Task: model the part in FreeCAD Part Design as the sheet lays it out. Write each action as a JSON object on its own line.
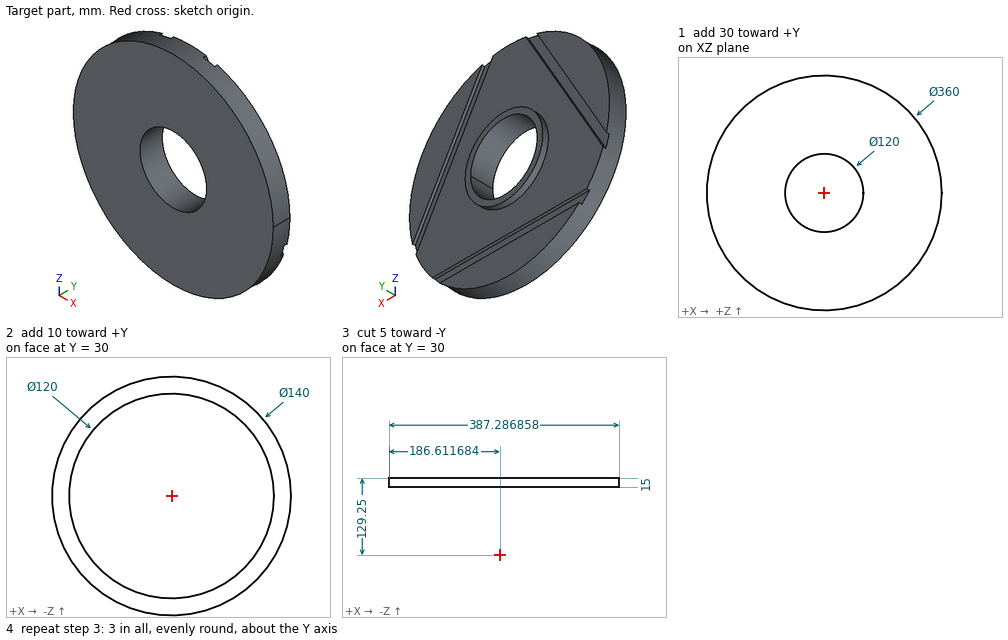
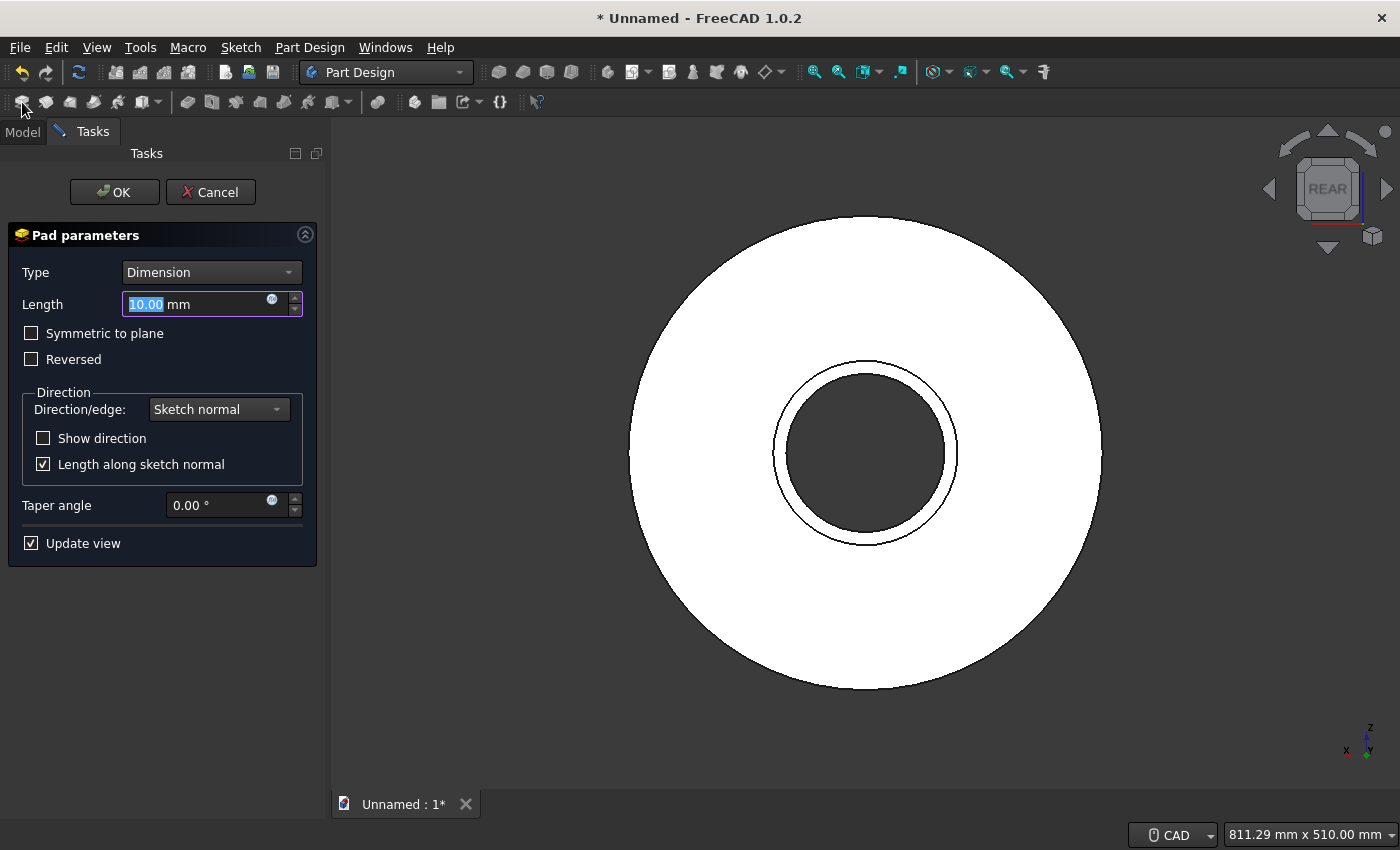
{"action": "type", "text": "10"}
{"action": "key", "text": "Tab"}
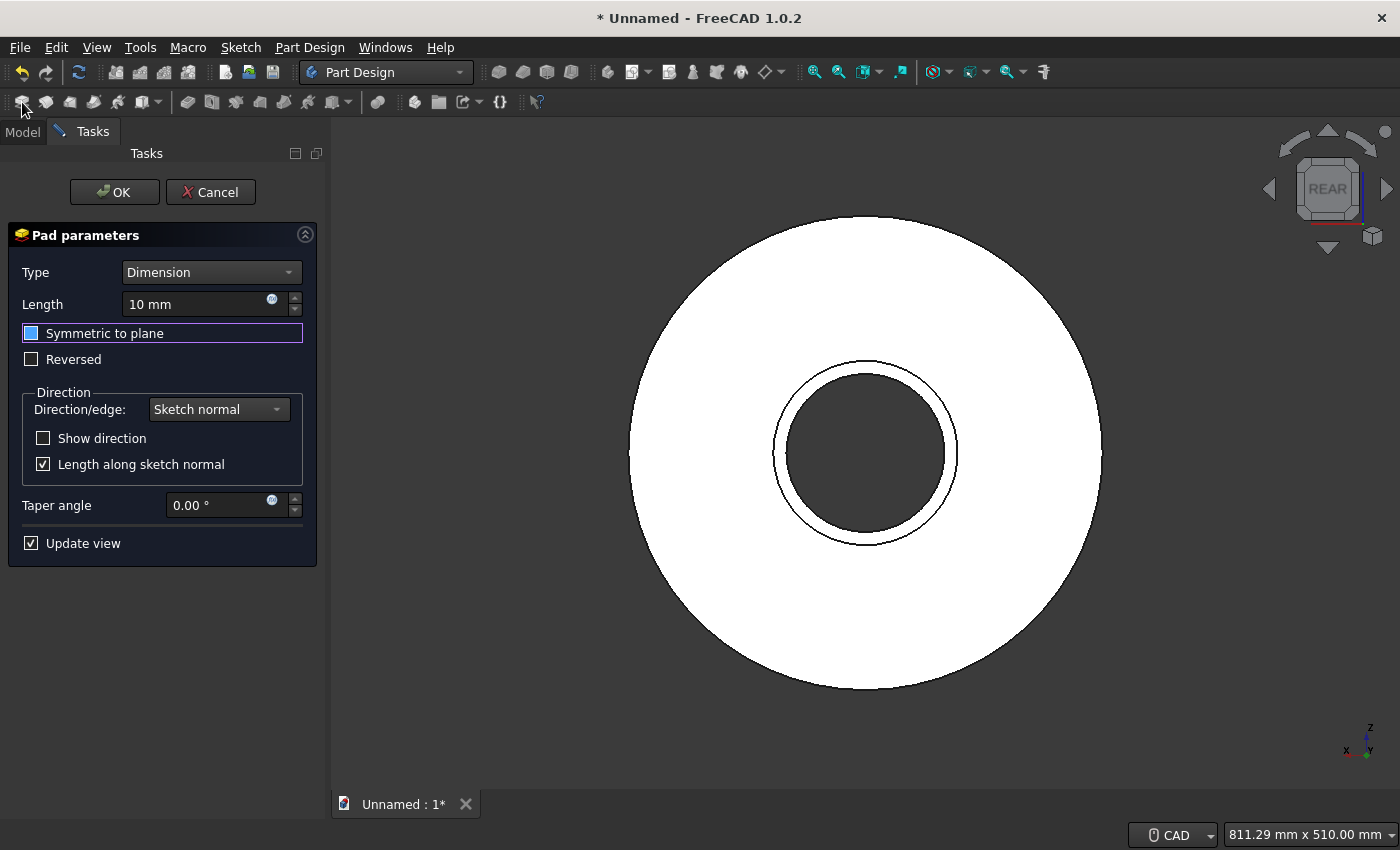
{"action": "left_click", "coordinate": [115, 192]}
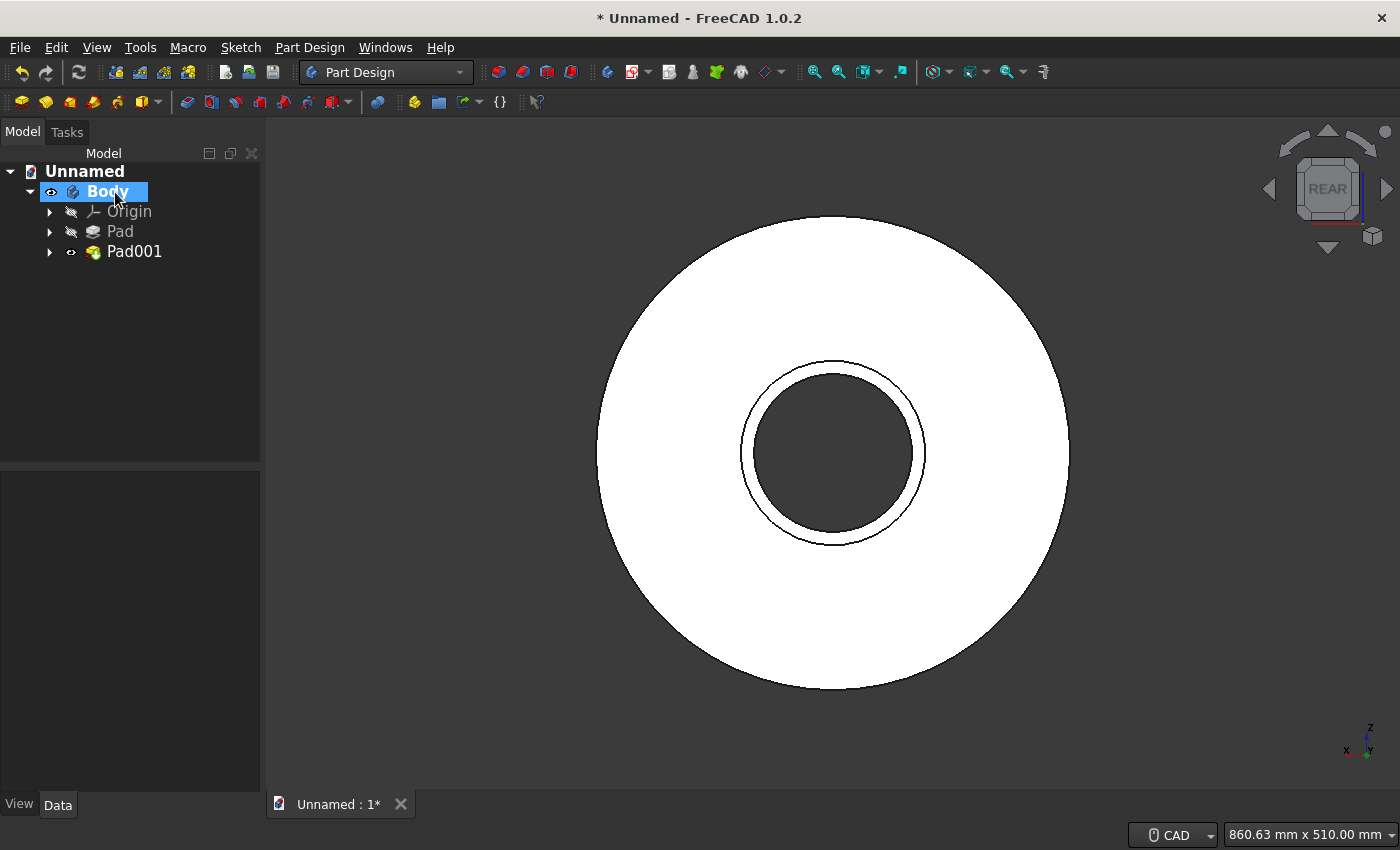
{"action": "left_click", "coordinate": [901, 588]}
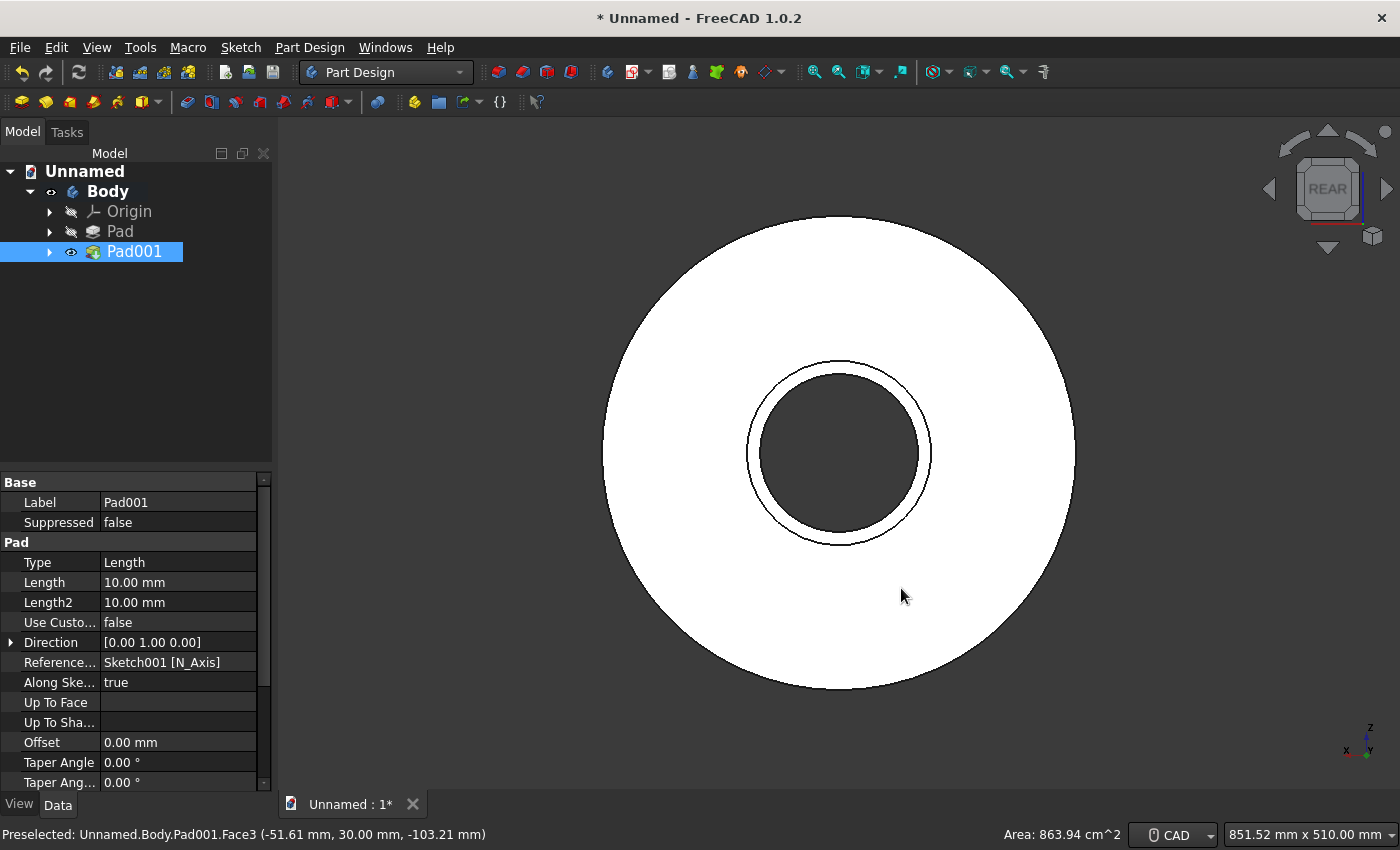
{"action": "left_click", "coordinate": [632, 72]}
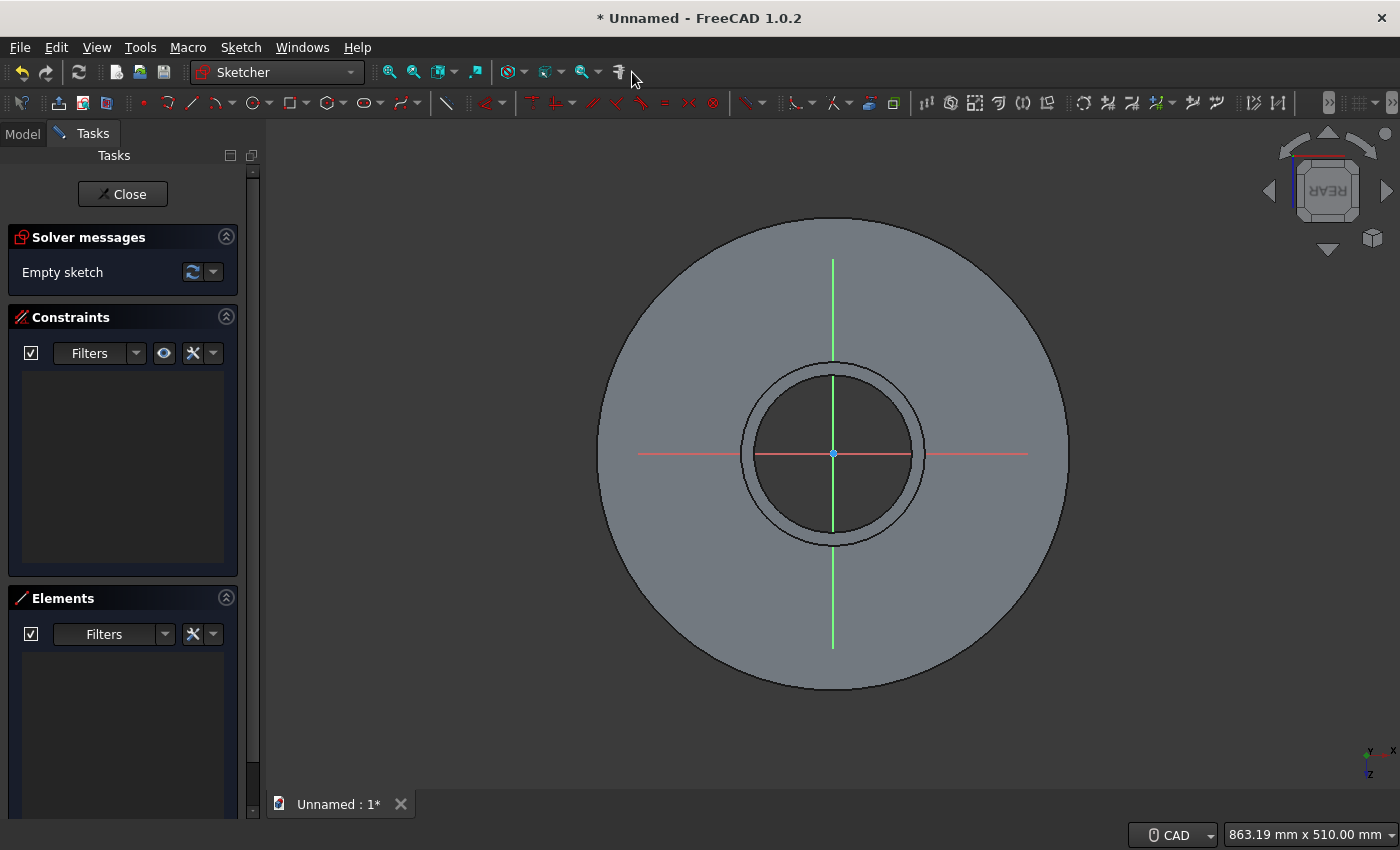
{"action": "left_click", "coordinate": [290, 104]}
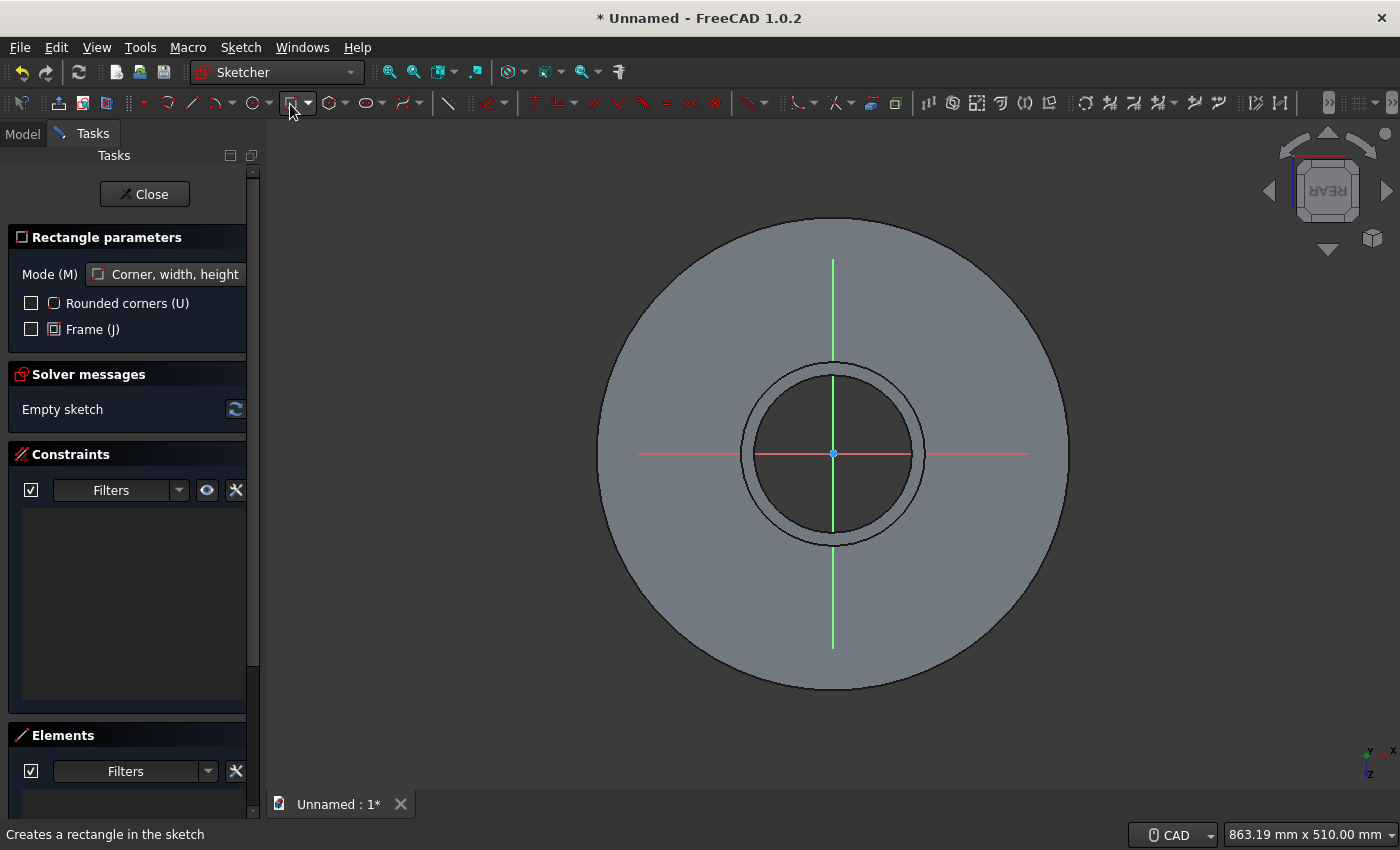
{"action": "left_click", "coordinate": [588, 284]}
{"action": "mouse_move", "coordinate": [1097, 304]}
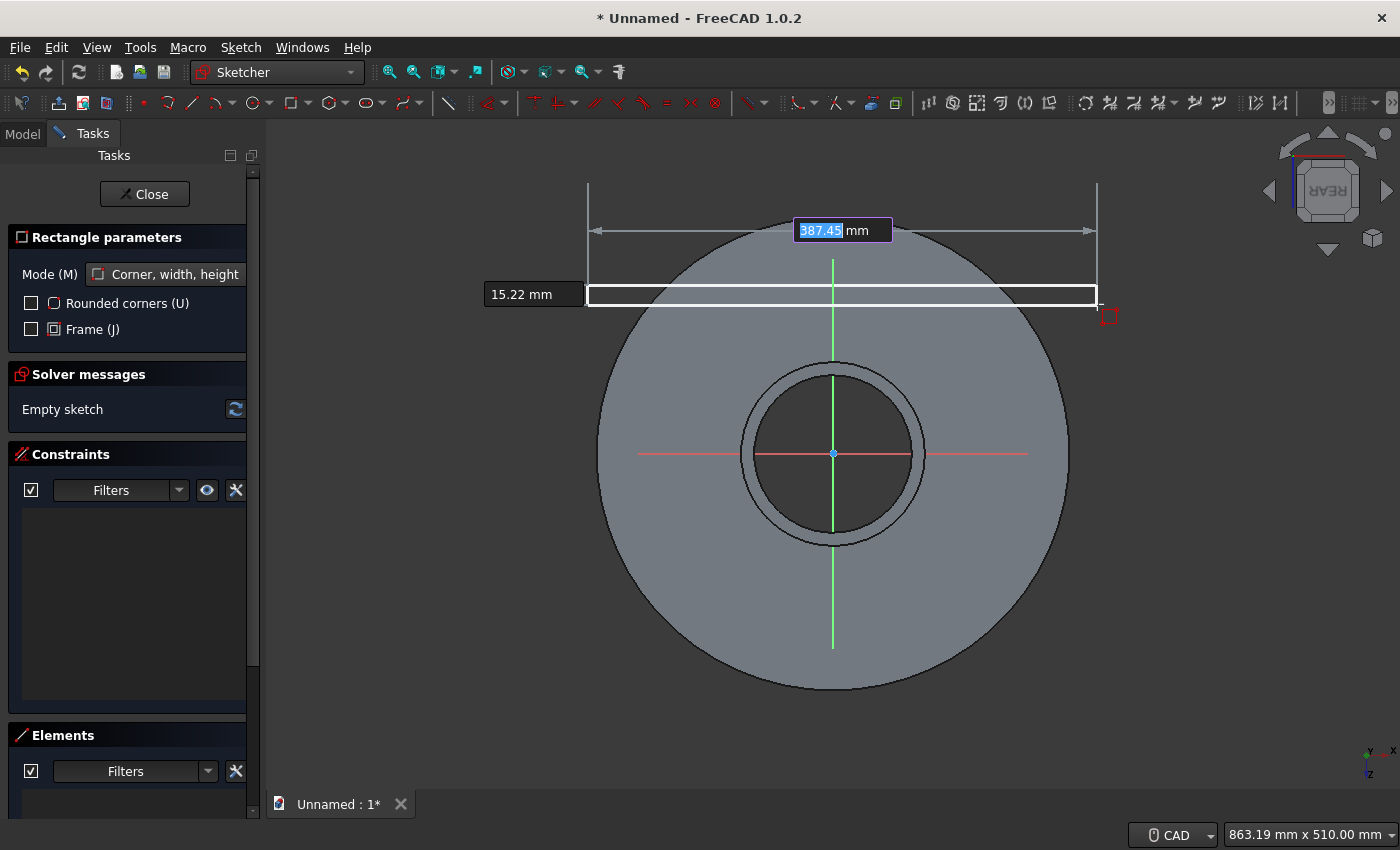
{"action": "type", "text": "387.286858"}
{"action": "key", "text": "Tab"}
{"action": "type", "text": "15"}
{"action": "key", "text": "Return"}
{"action": "key", "text": "Escape"}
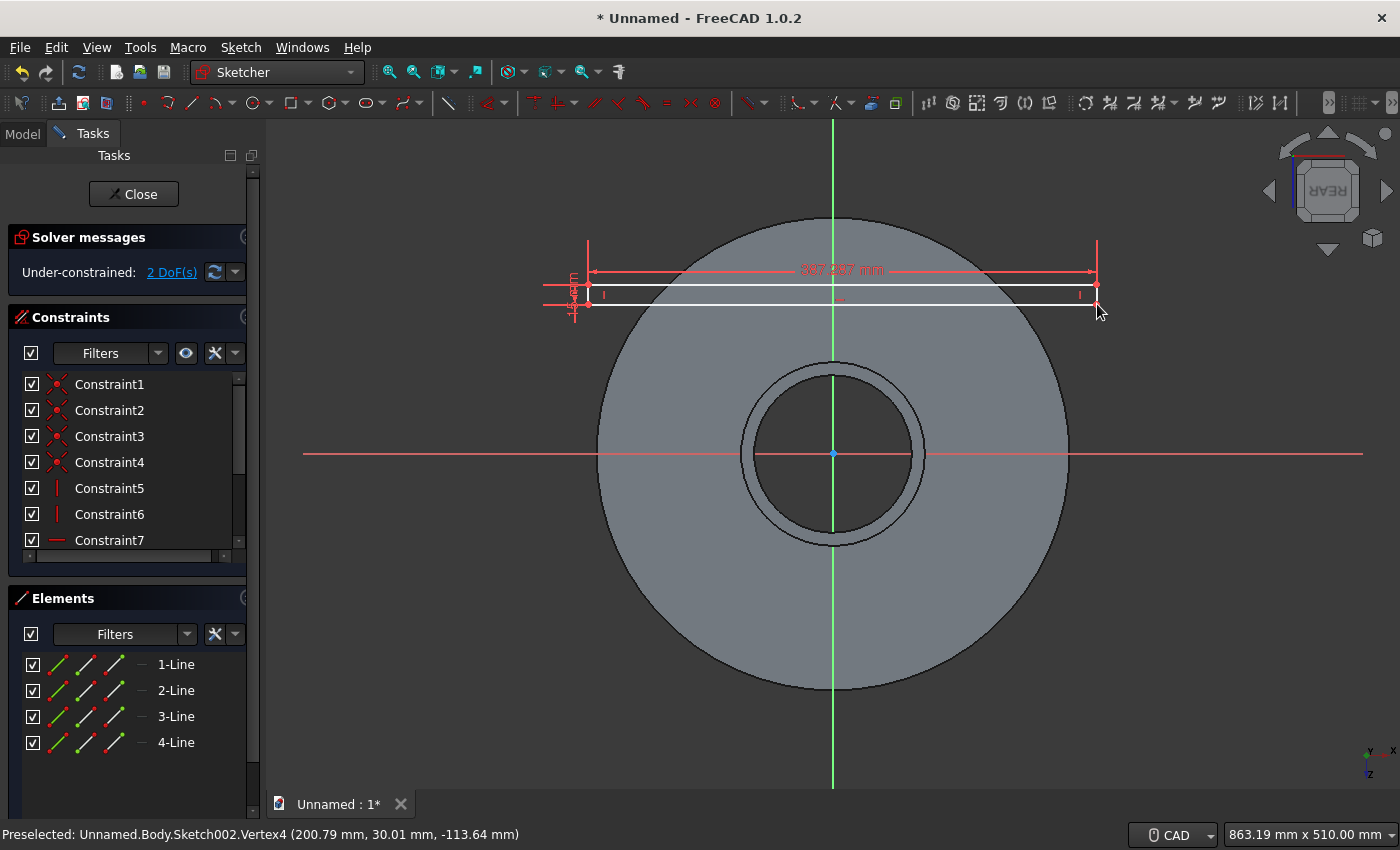
{"action": "left_click", "coordinate": [588, 285]}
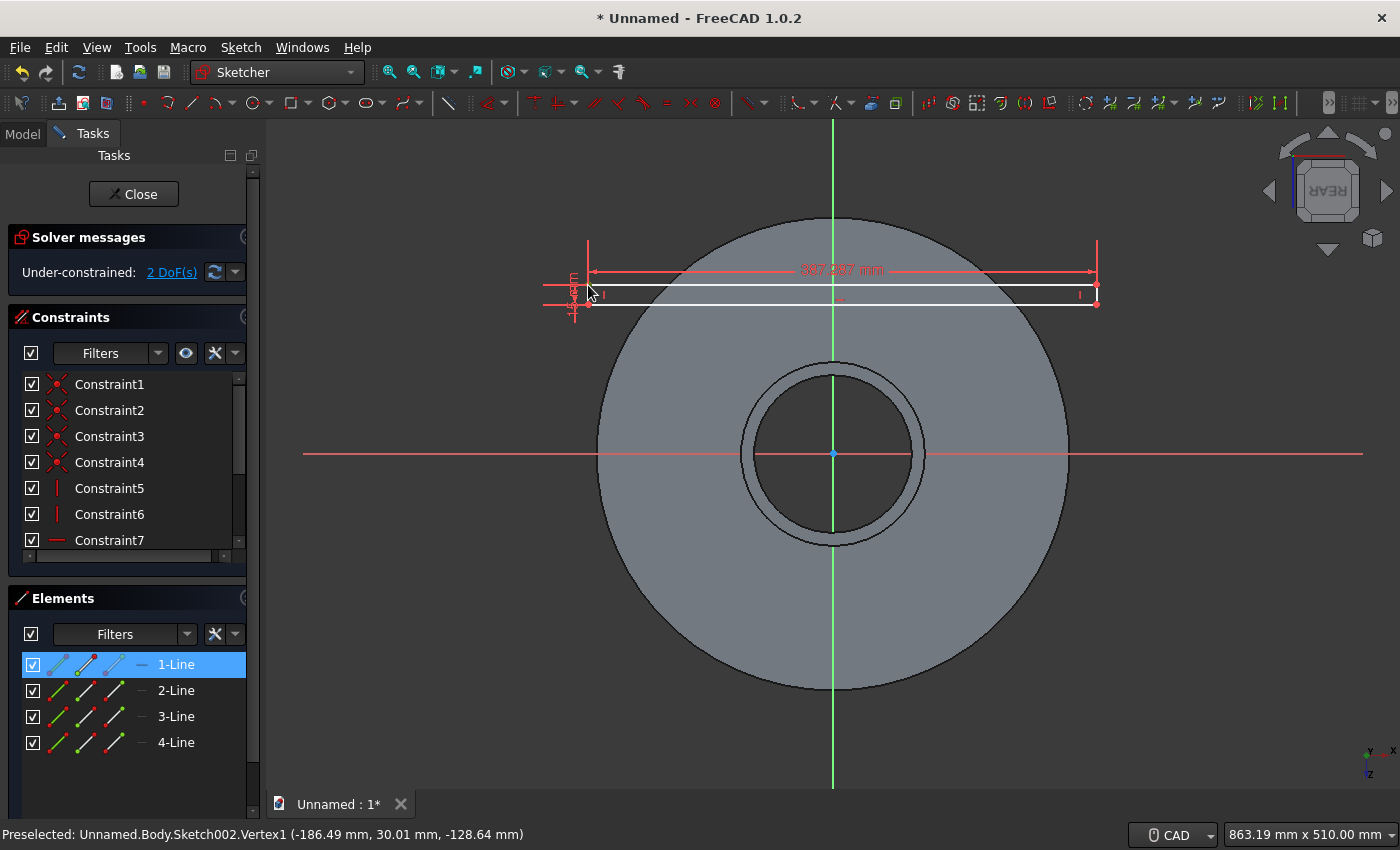
{"action": "key", "text": "i"}